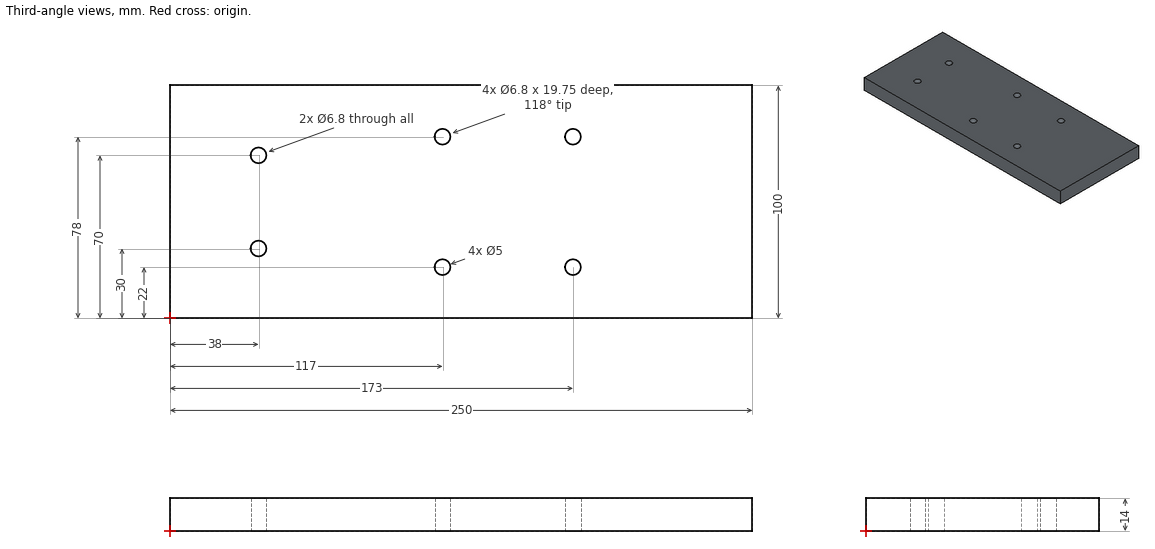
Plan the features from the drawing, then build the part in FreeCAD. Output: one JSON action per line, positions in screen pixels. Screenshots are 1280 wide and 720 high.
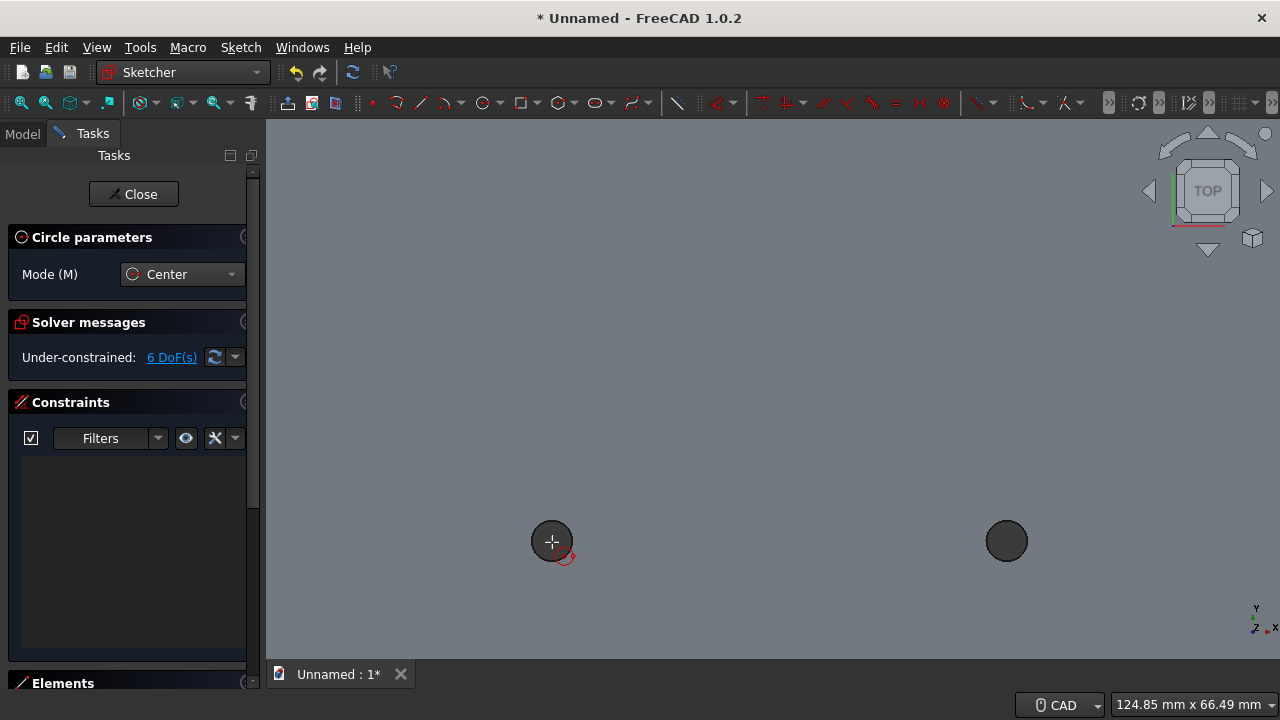
{"action": "left_click", "coordinate": [552, 541]}
{"action": "left_click", "coordinate": [572, 521]}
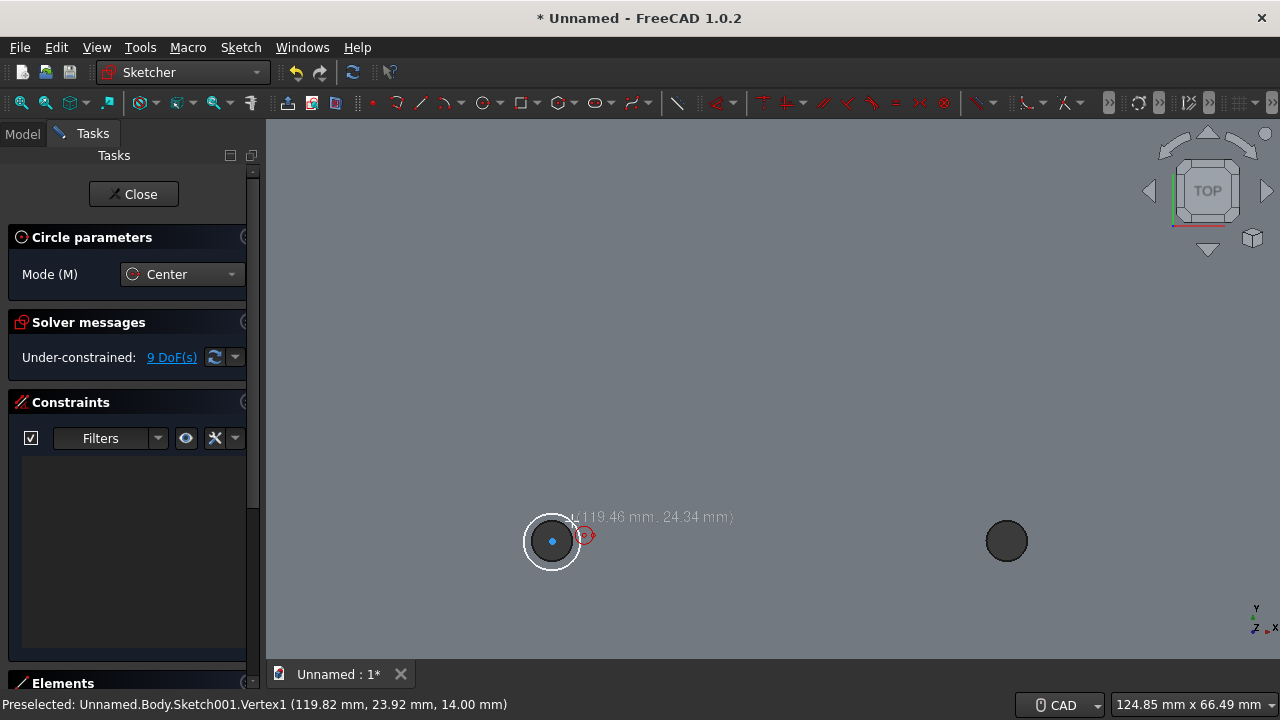
{"action": "left_click", "coordinate": [1007, 541]}
{"action": "left_click", "coordinate": [1026, 521]}
{"action": "key", "text": "Escape"}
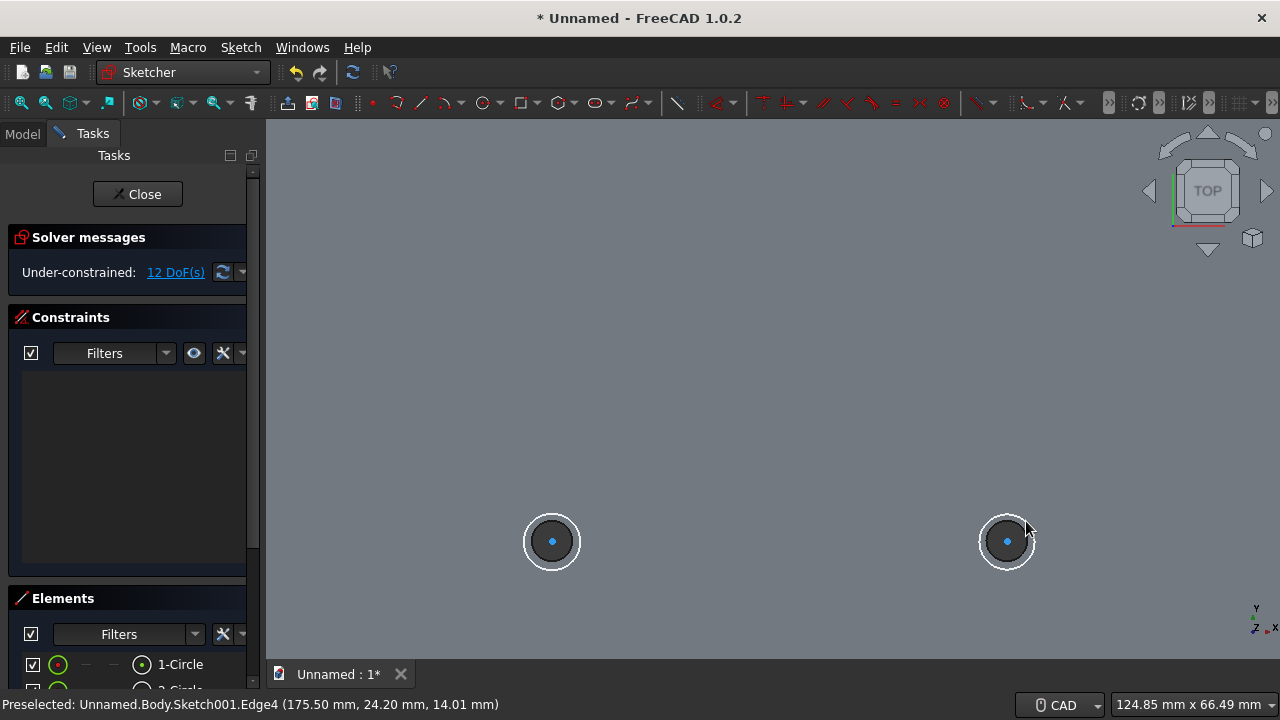
{"action": "scroll", "coordinate": [552, 542], "scroll_direction": "down", "scroll_amount": 2}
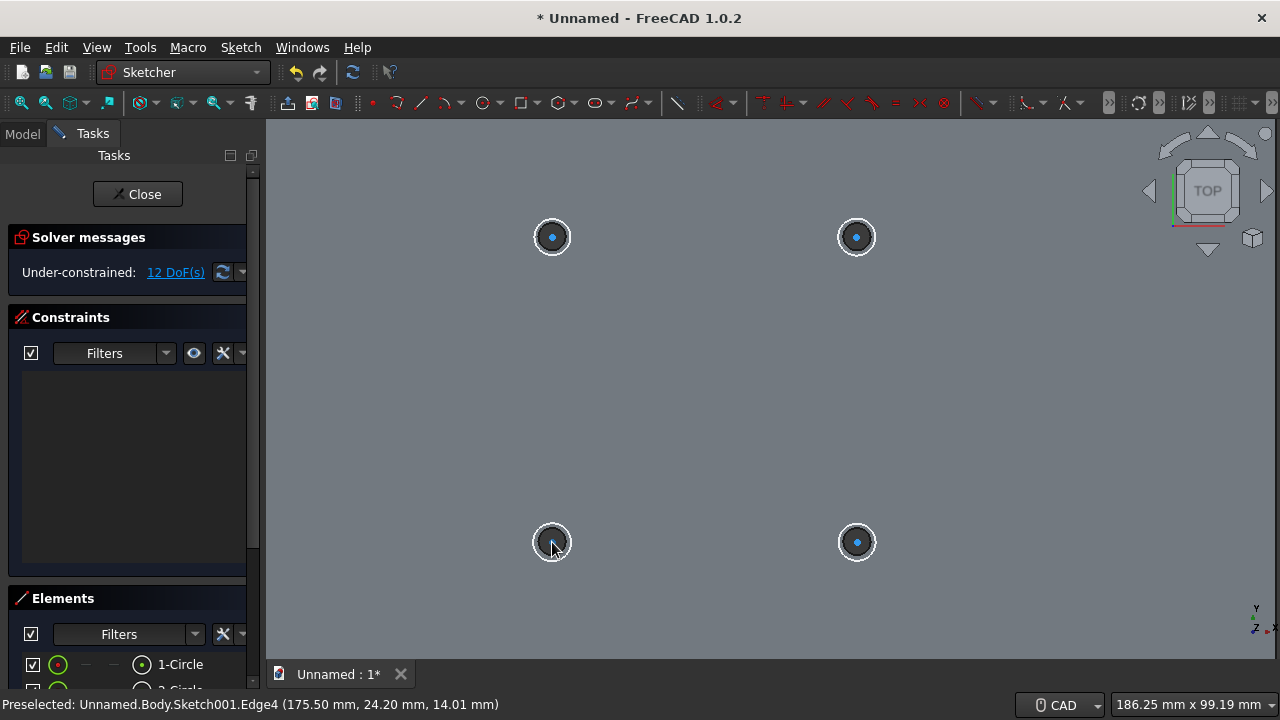
{"action": "left_click", "coordinate": [565, 224]}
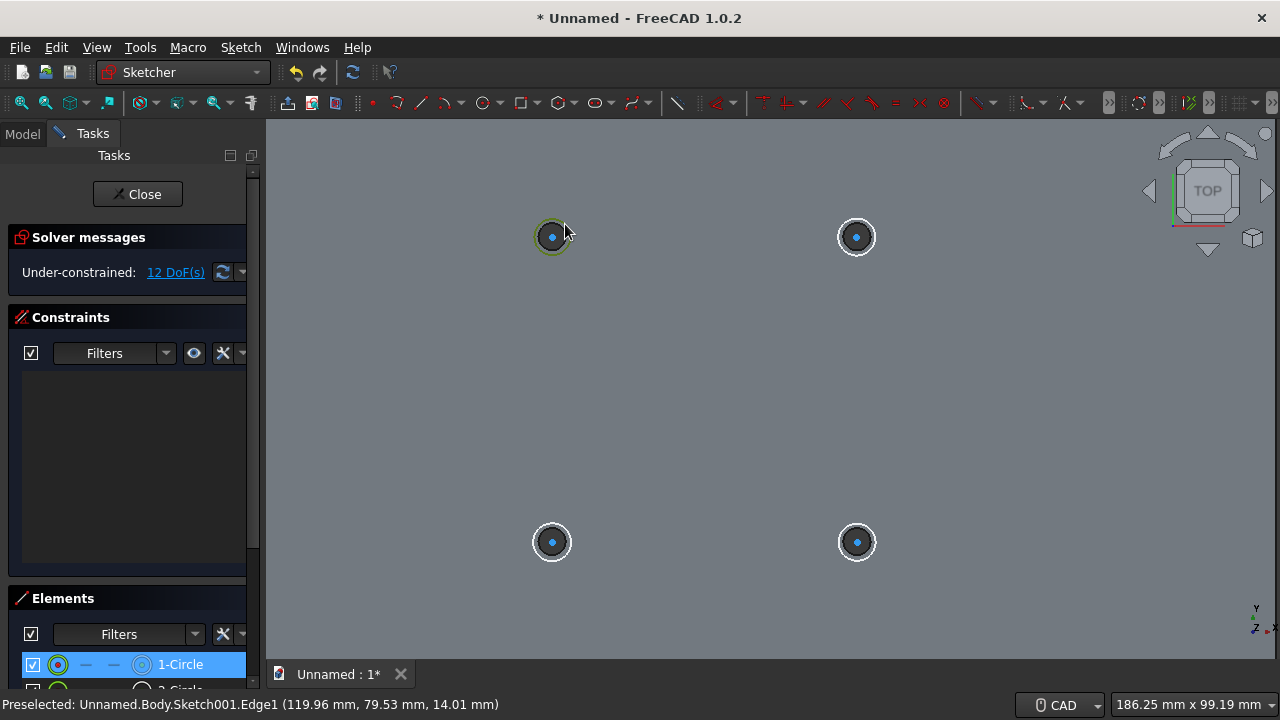
{"action": "left_click", "coordinate": [870, 224]}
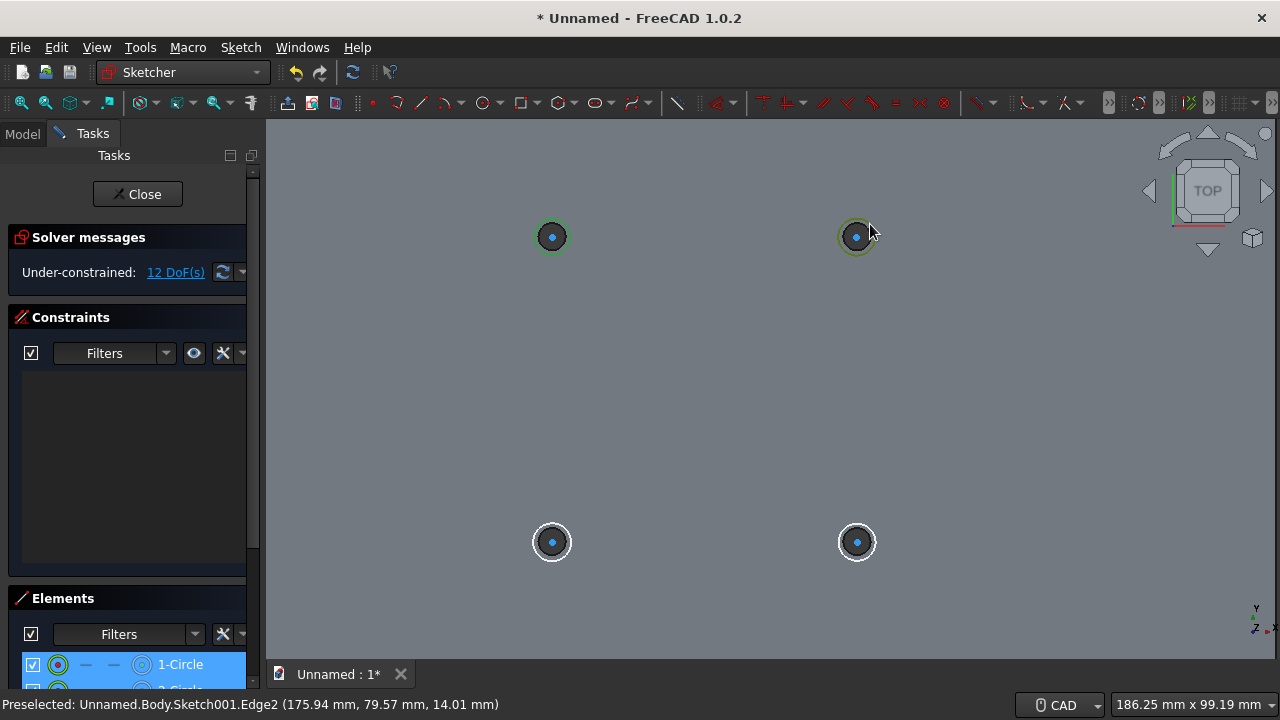
{"action": "left_click", "coordinate": [565, 529]}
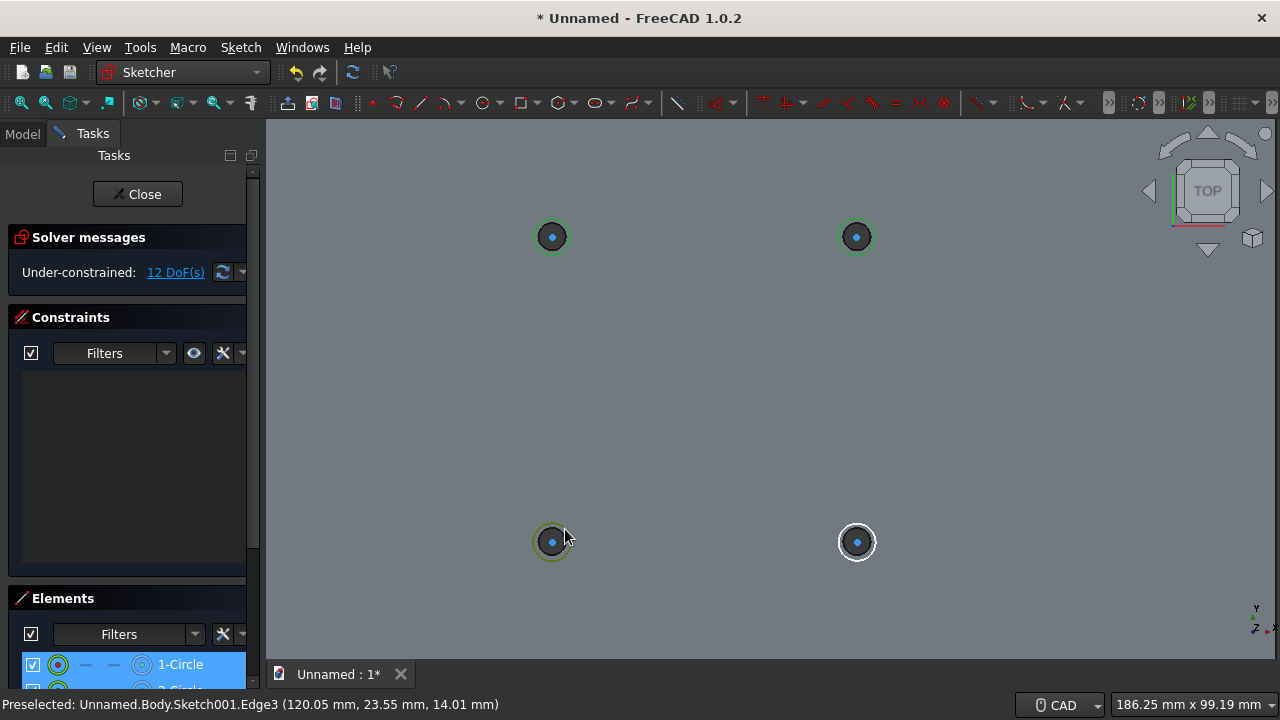
{"action": "left_click", "coordinate": [870, 529]}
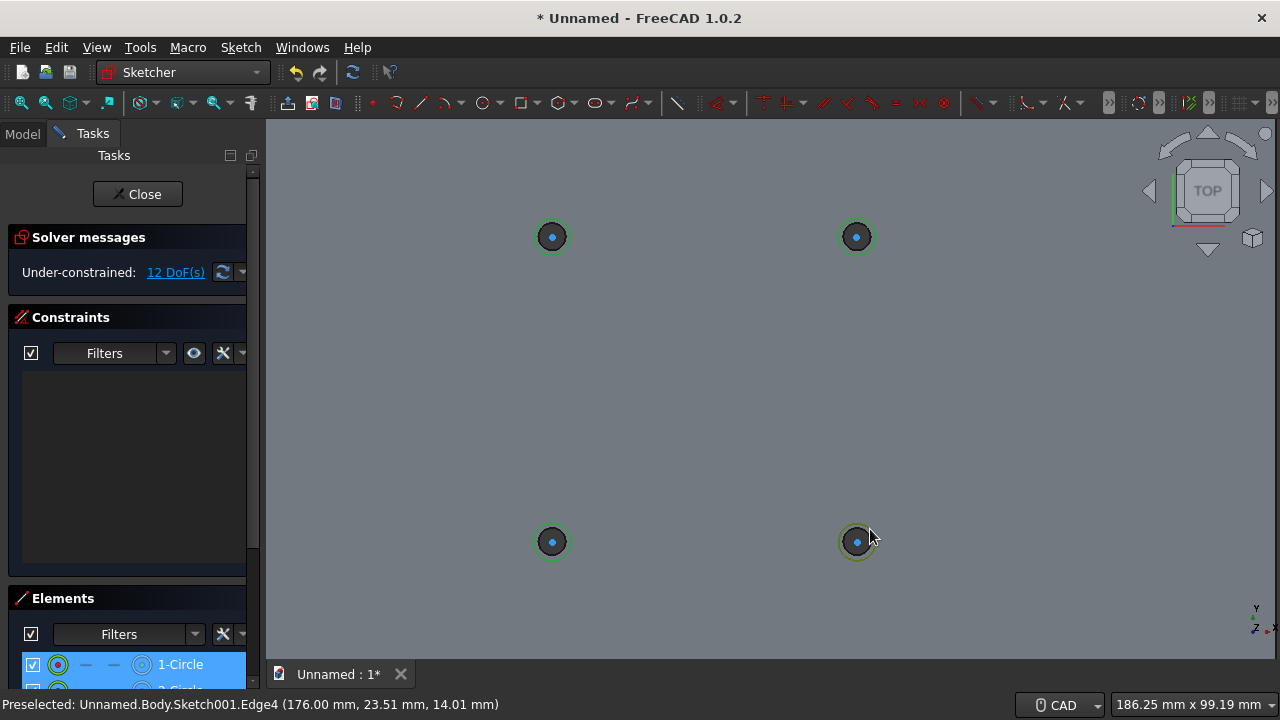
{"action": "key", "text": "e"}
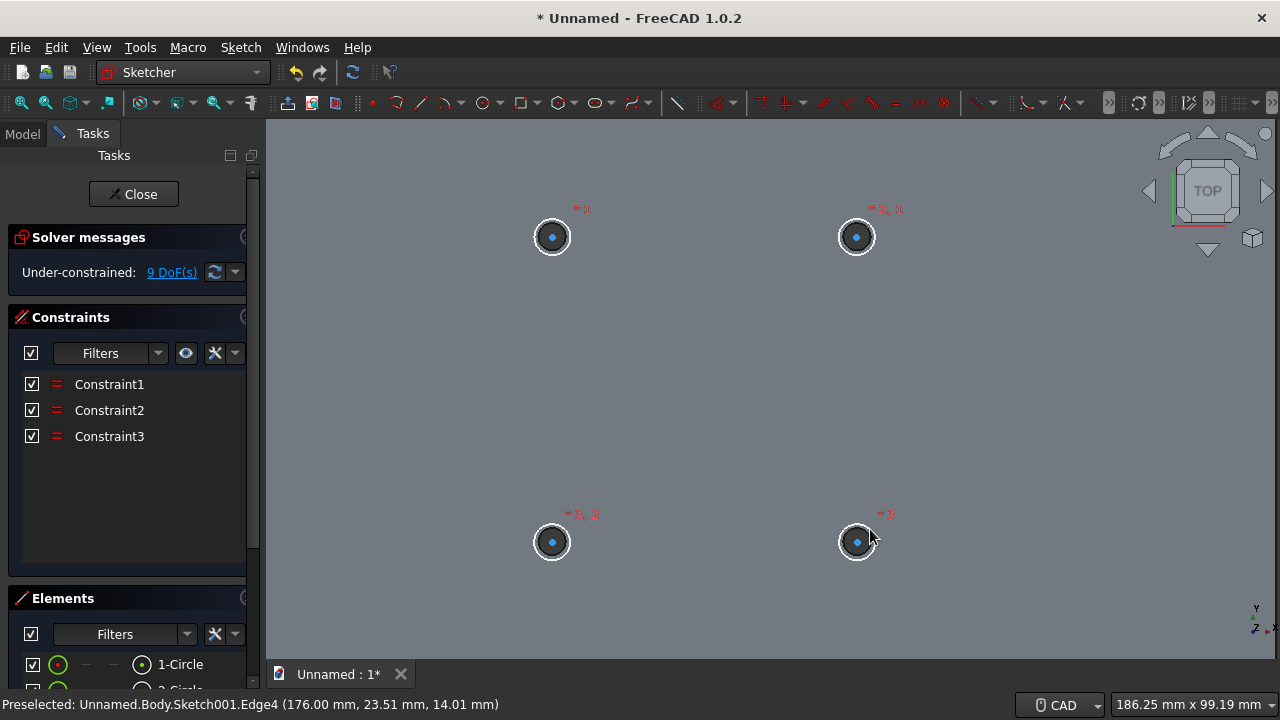
{"action": "left_click", "coordinate": [716, 104]}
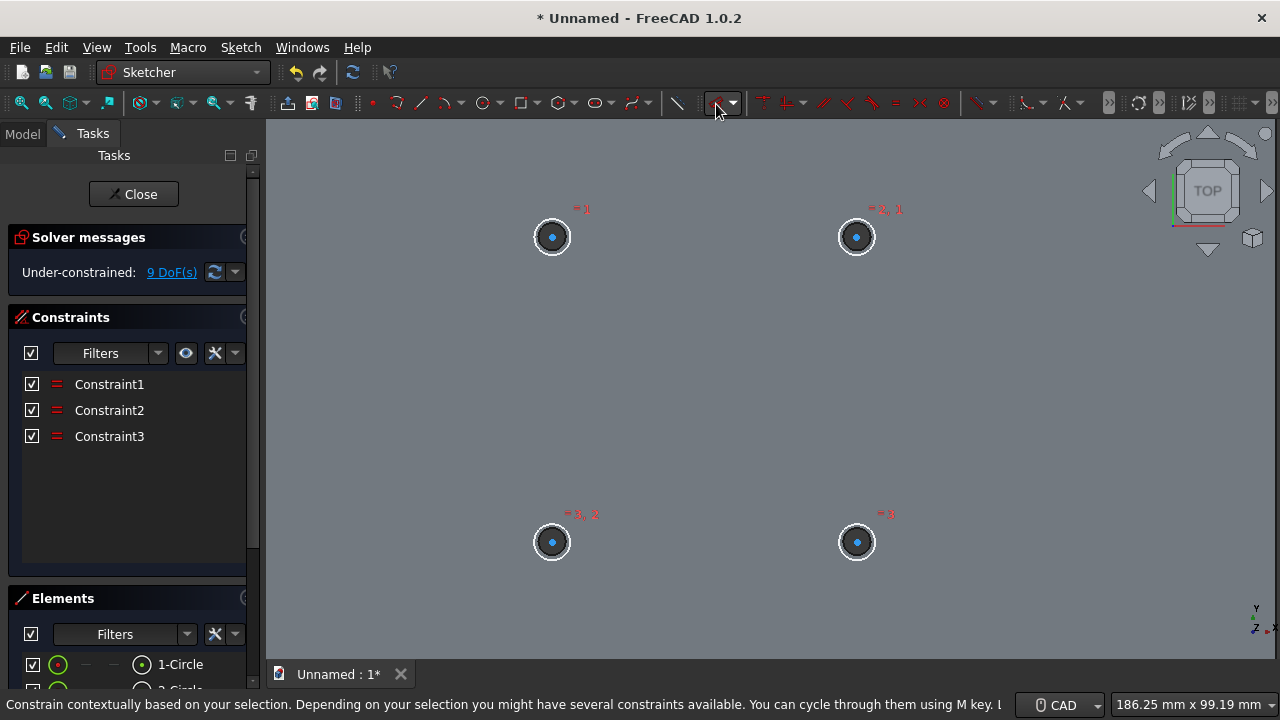
{"action": "left_click", "coordinate": [565, 224]}
{"action": "left_click", "coordinate": [587, 201]}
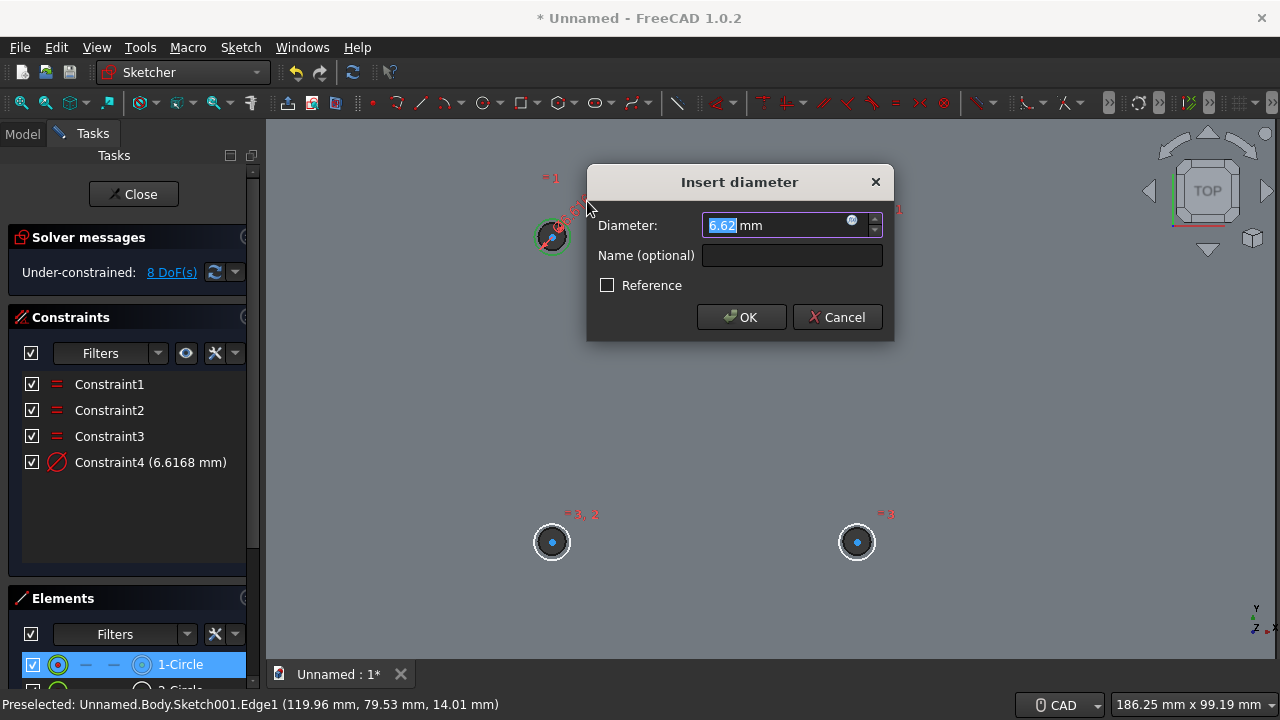
{"action": "type", "text": "6.8"}
{"action": "key", "text": "Return"}